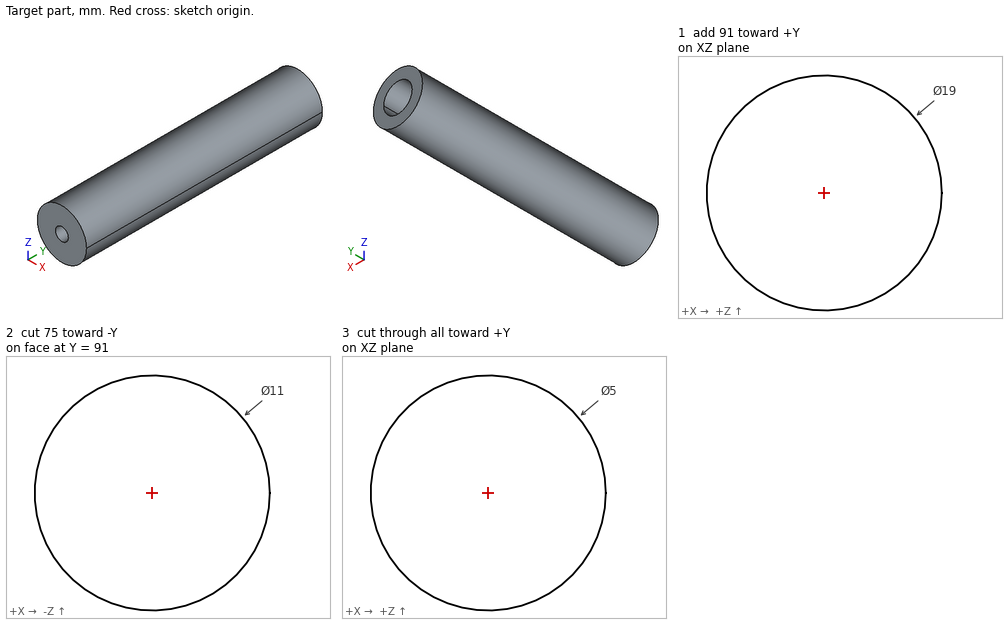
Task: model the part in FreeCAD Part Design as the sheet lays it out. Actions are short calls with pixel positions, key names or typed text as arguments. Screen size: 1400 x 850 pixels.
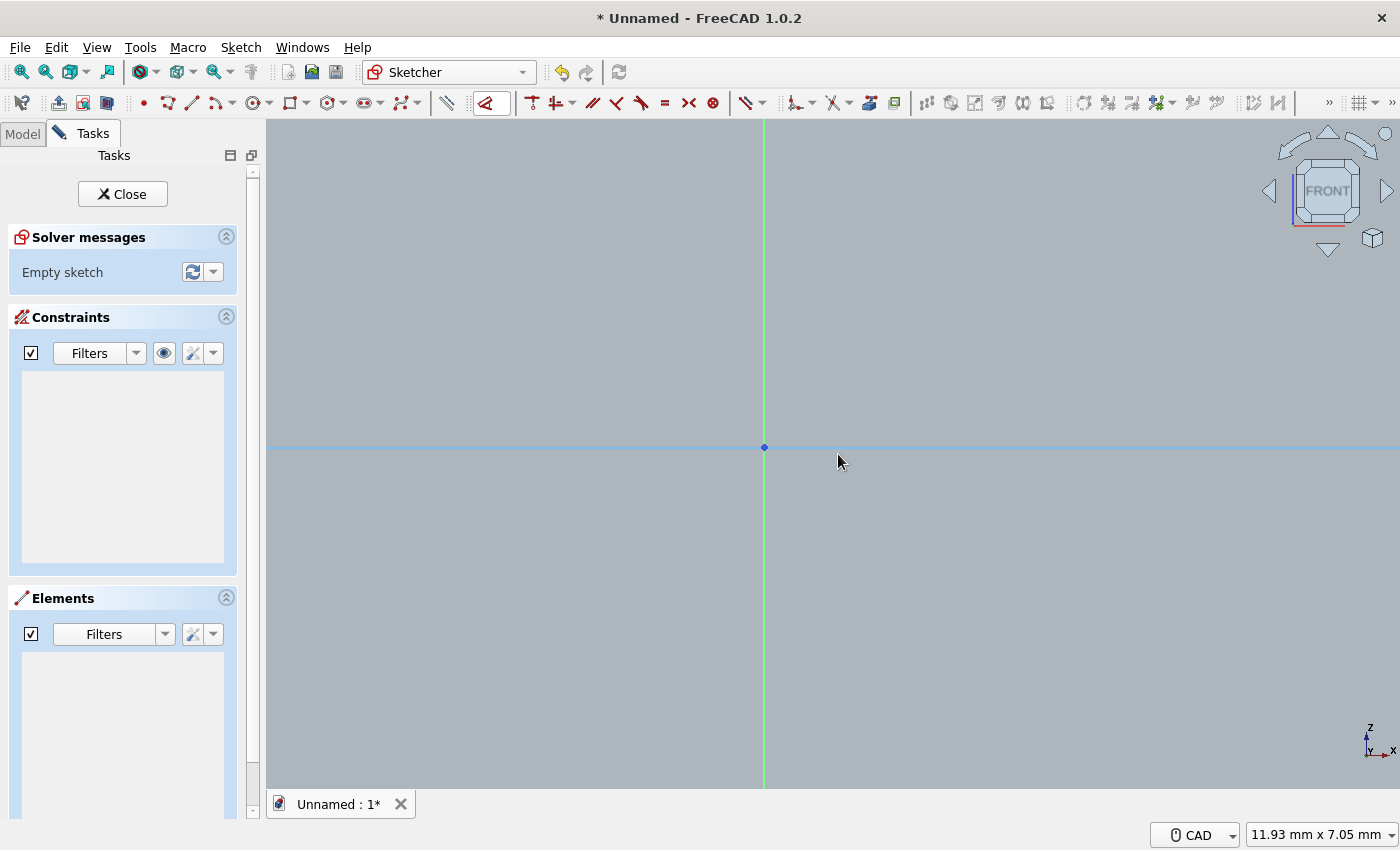
key(g)
key(c)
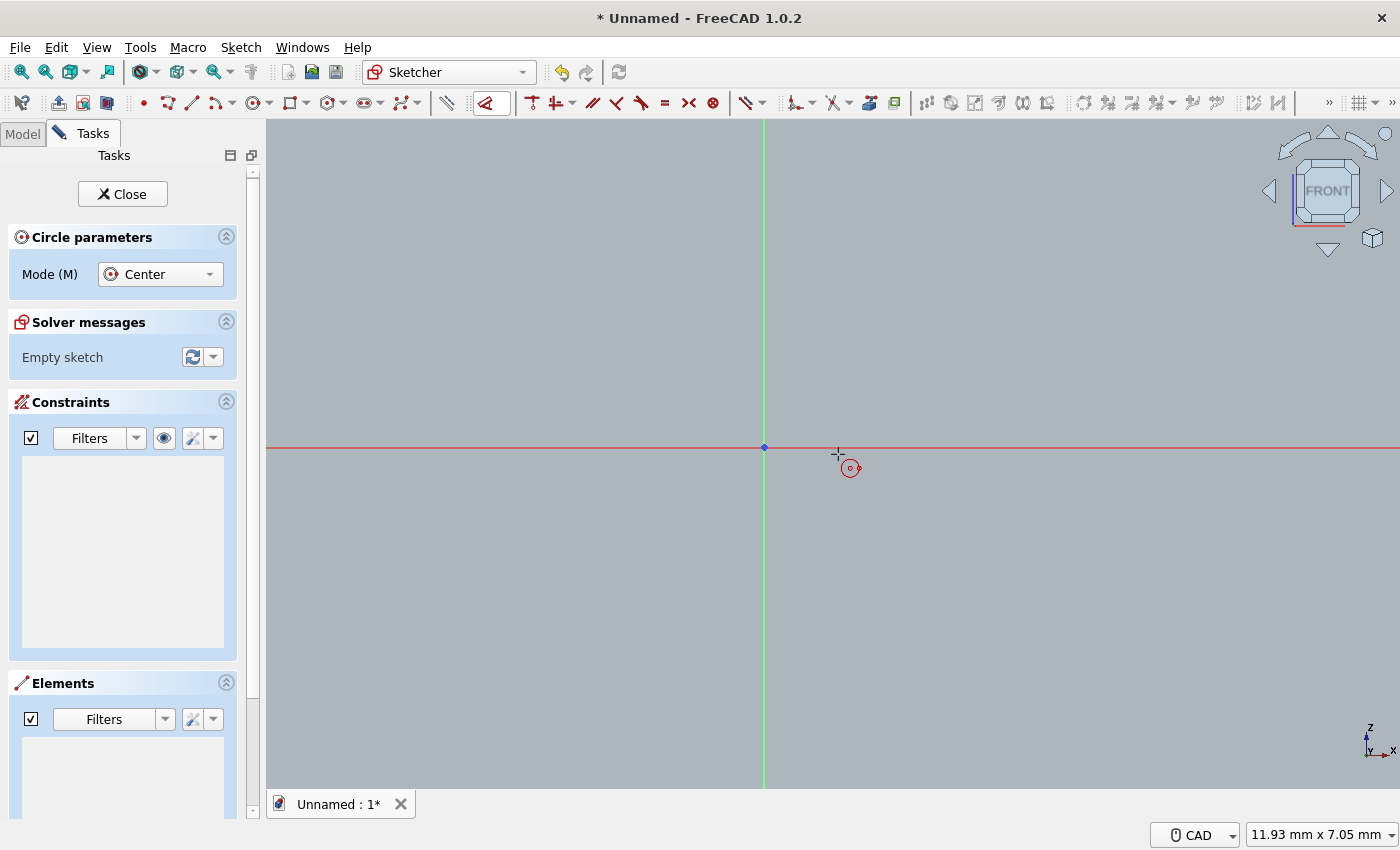
click(764, 448)
click(932, 280)
key(Escape)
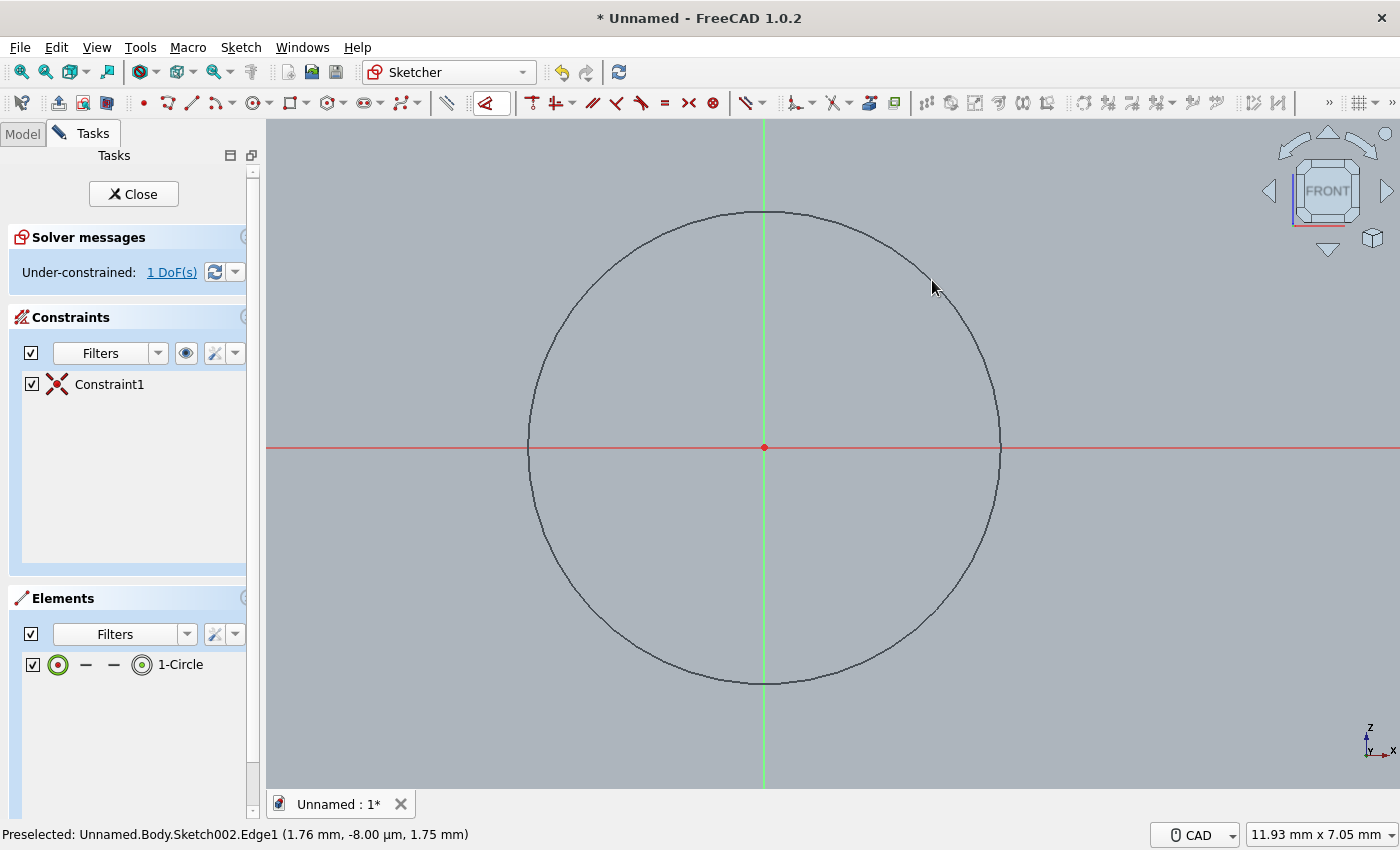
click(931, 280)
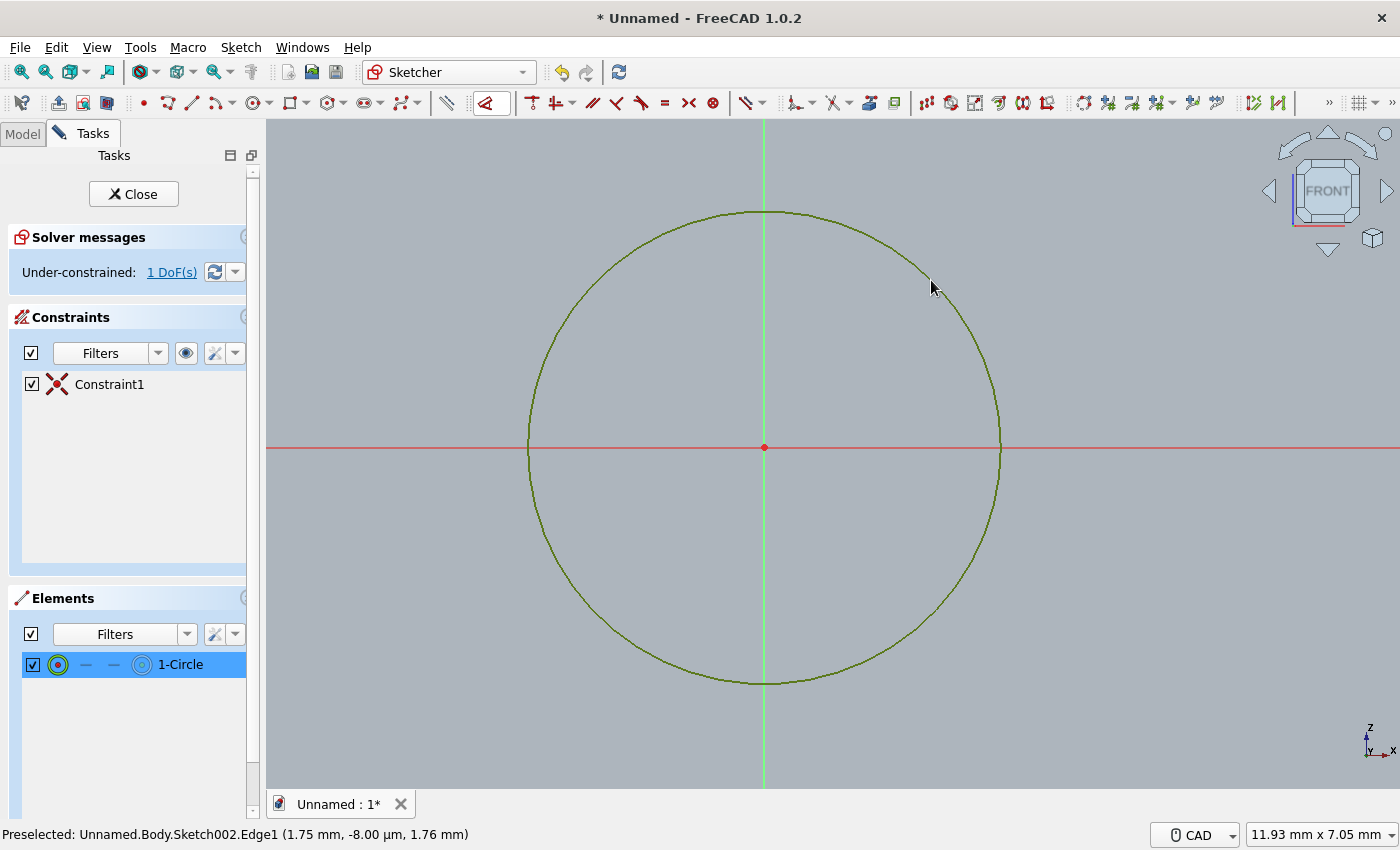
key(k)
key(o)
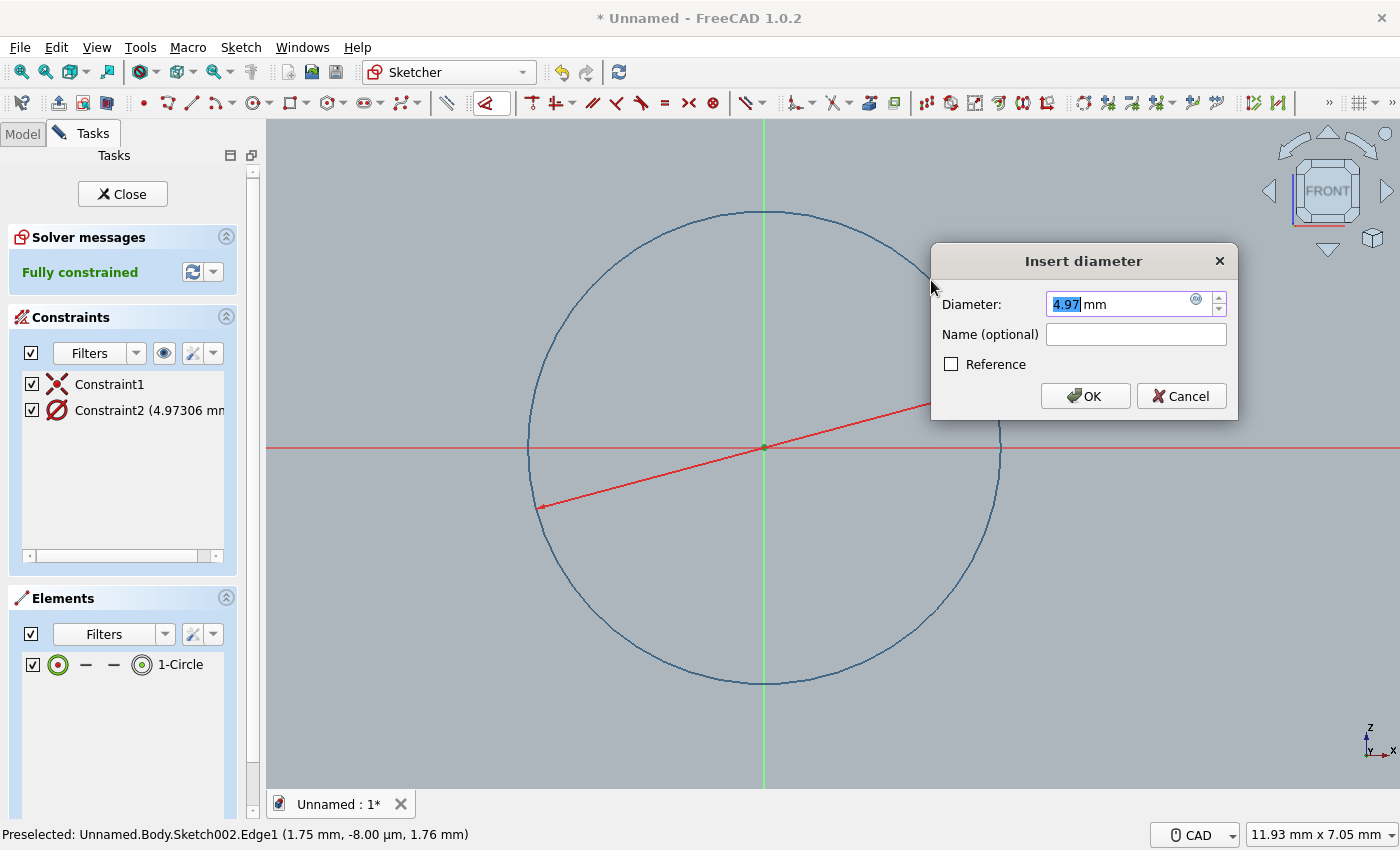
text(5)
key(Return)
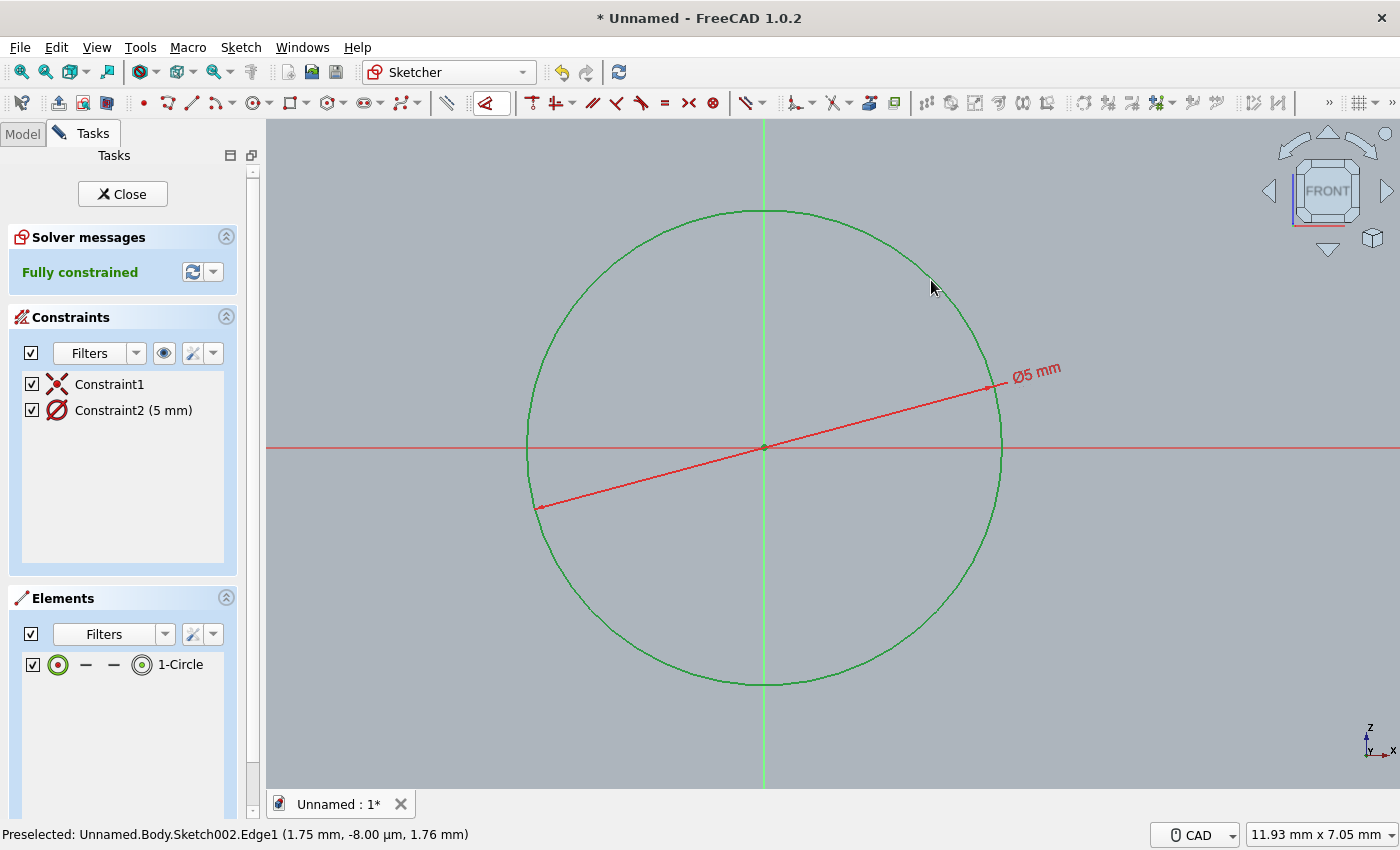
click(123, 194)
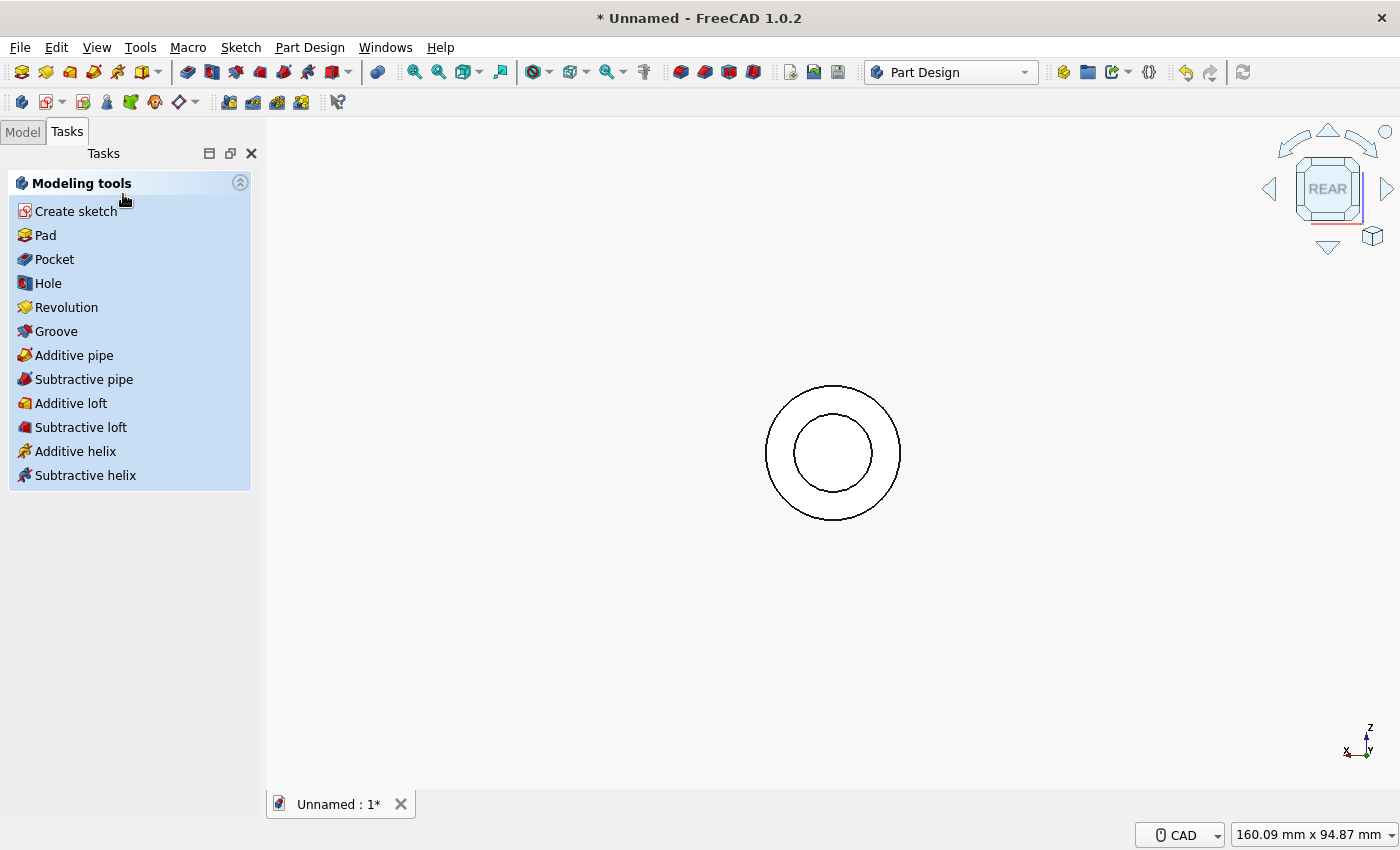
click(188, 72)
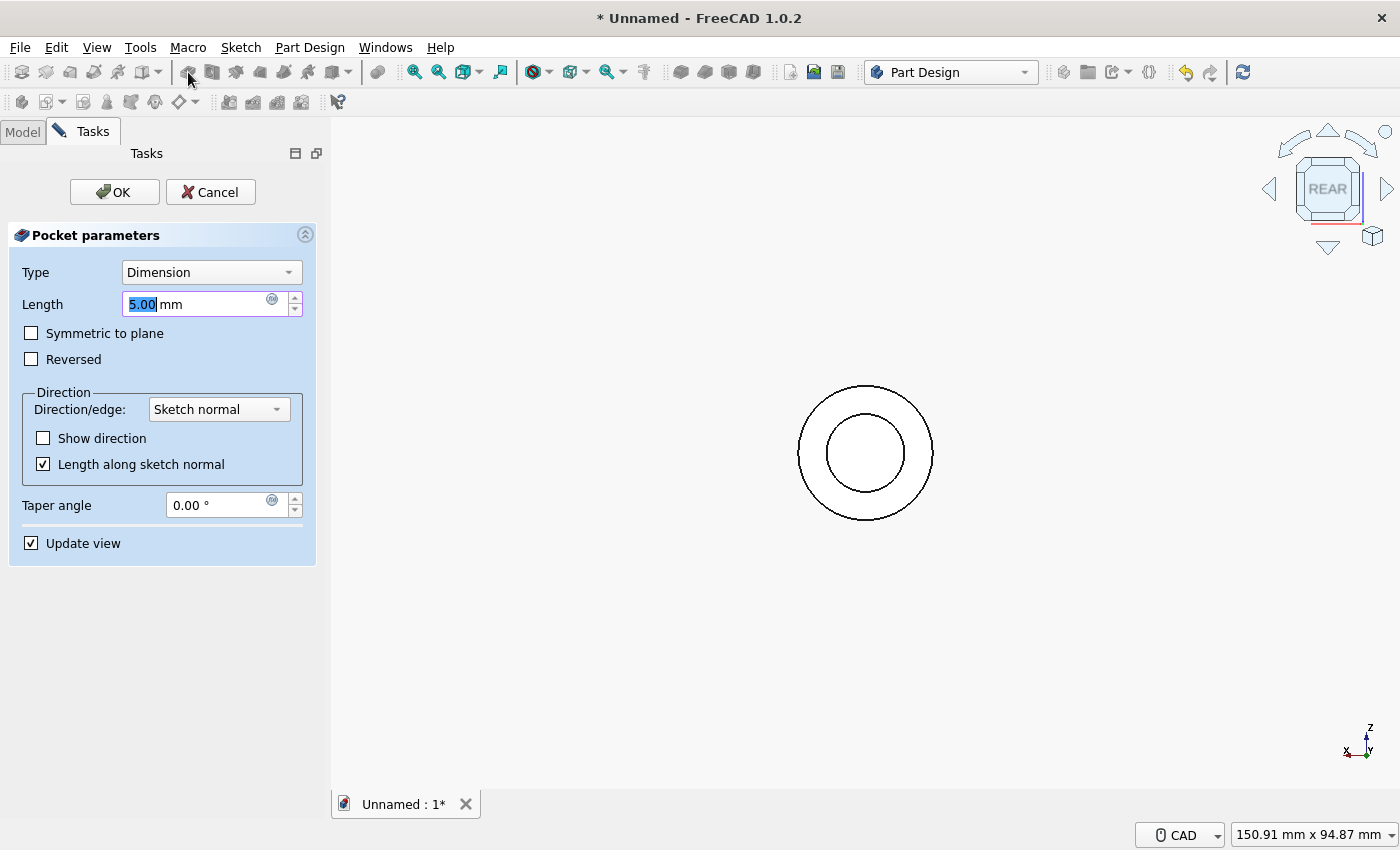
click(212, 272)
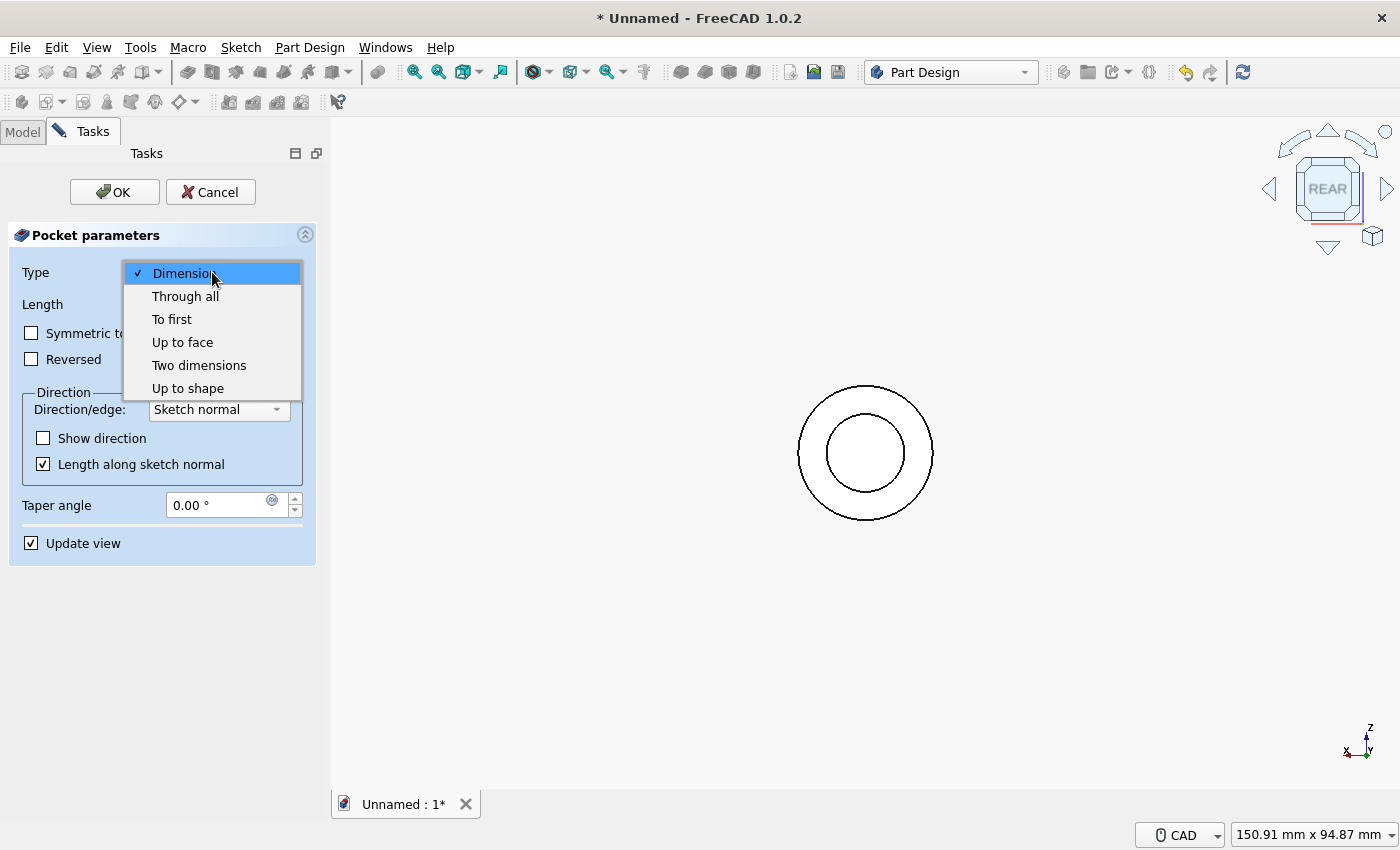
click(212, 296)